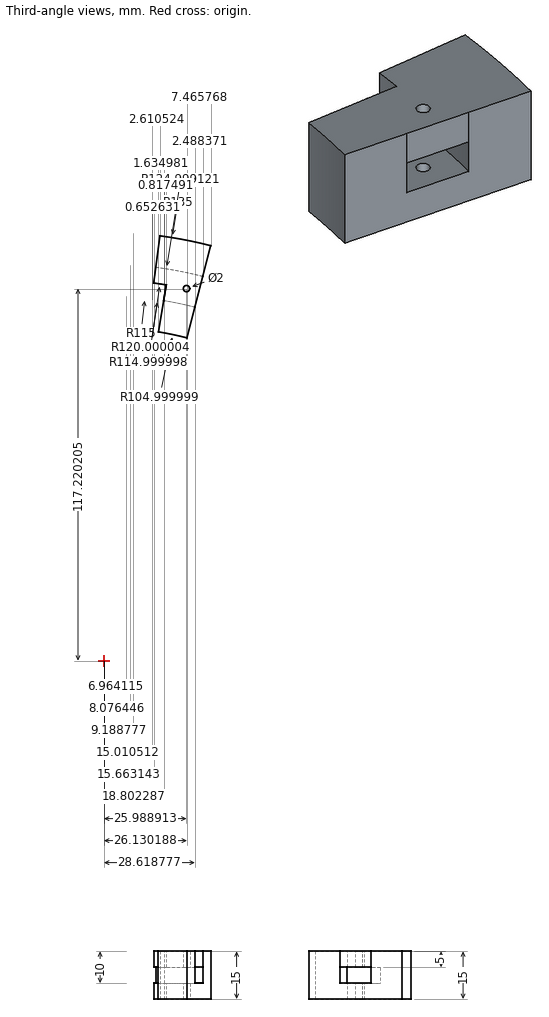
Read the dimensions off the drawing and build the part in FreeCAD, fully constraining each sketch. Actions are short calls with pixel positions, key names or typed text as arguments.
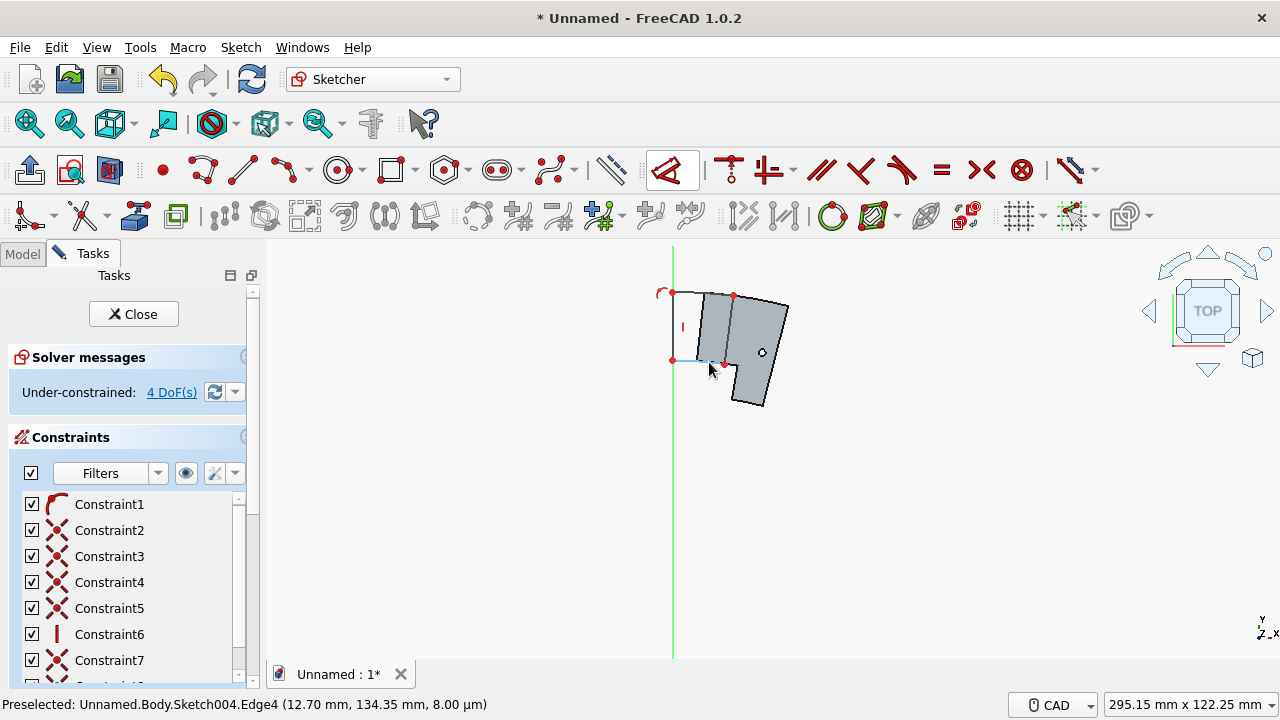
click(709, 362)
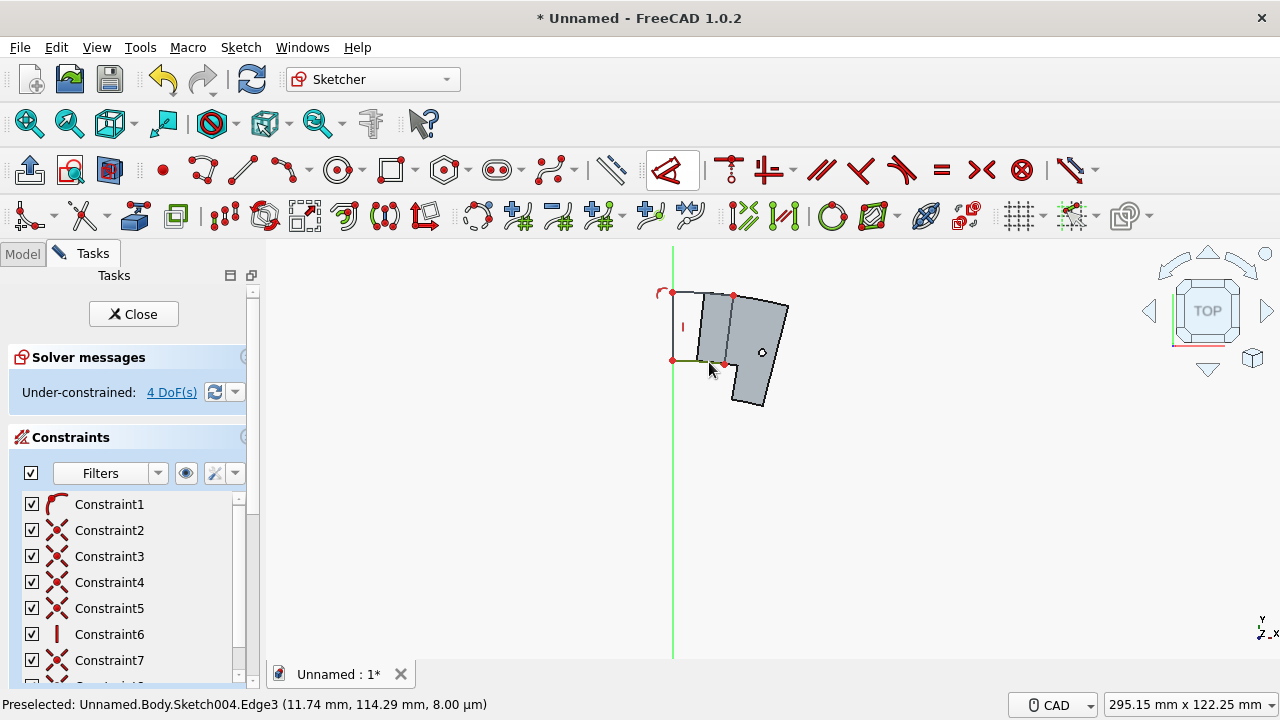
click(694, 170)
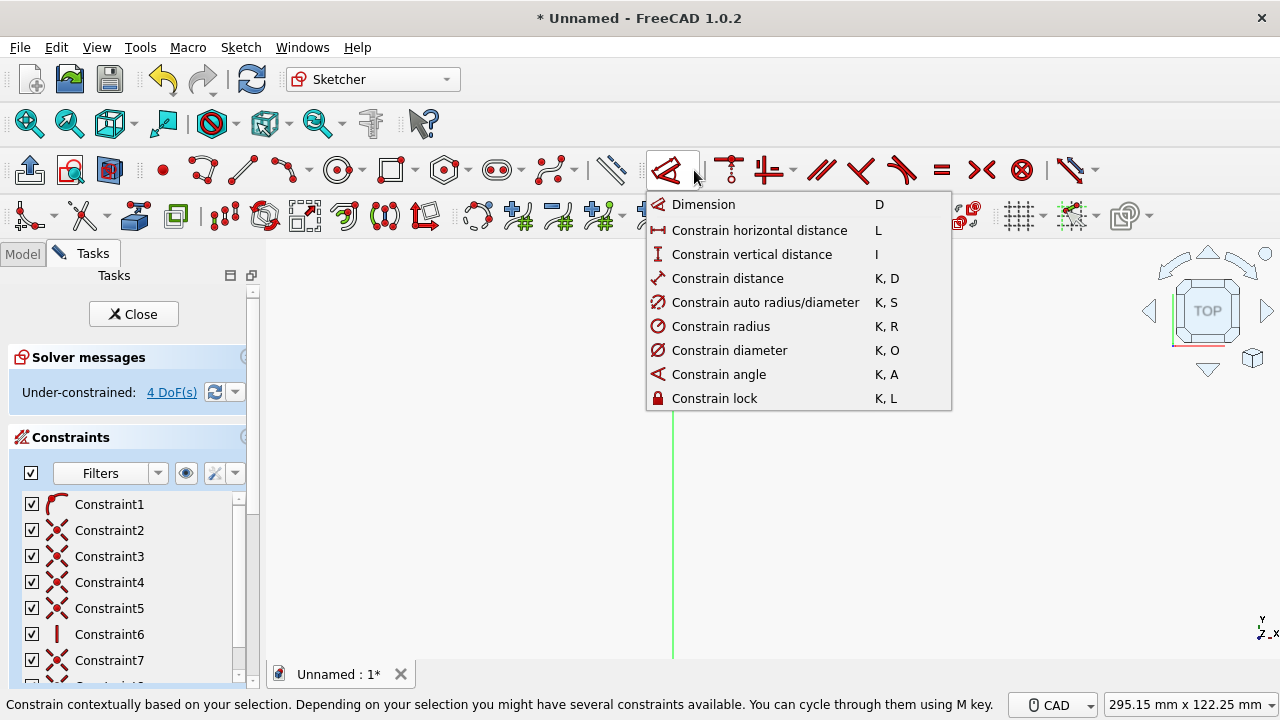
click(799, 326)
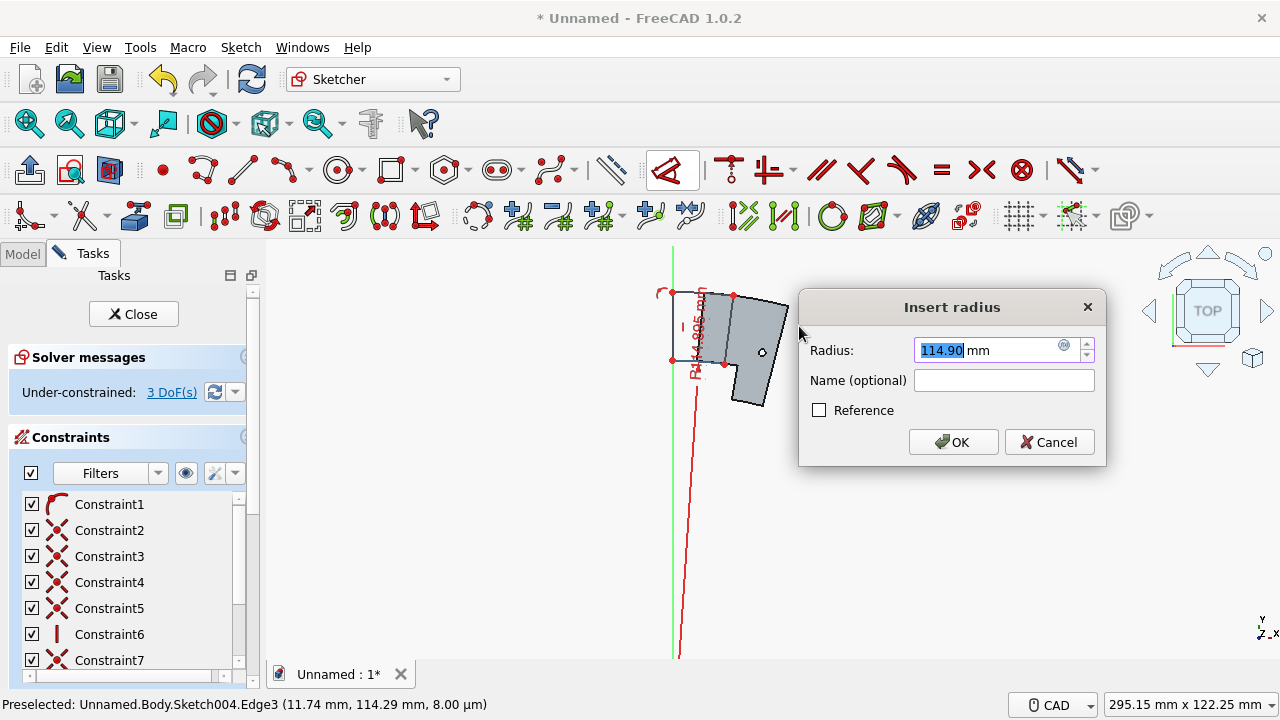
text(115)
key(Return)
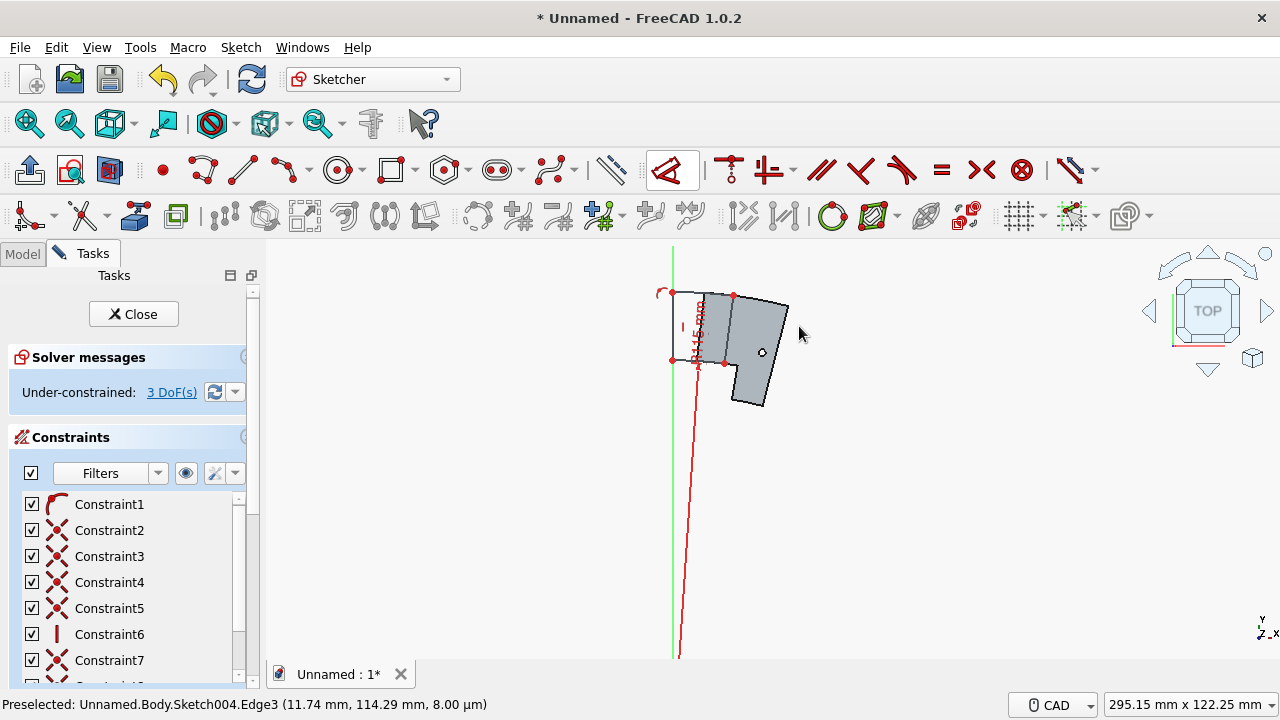
click(715, 294)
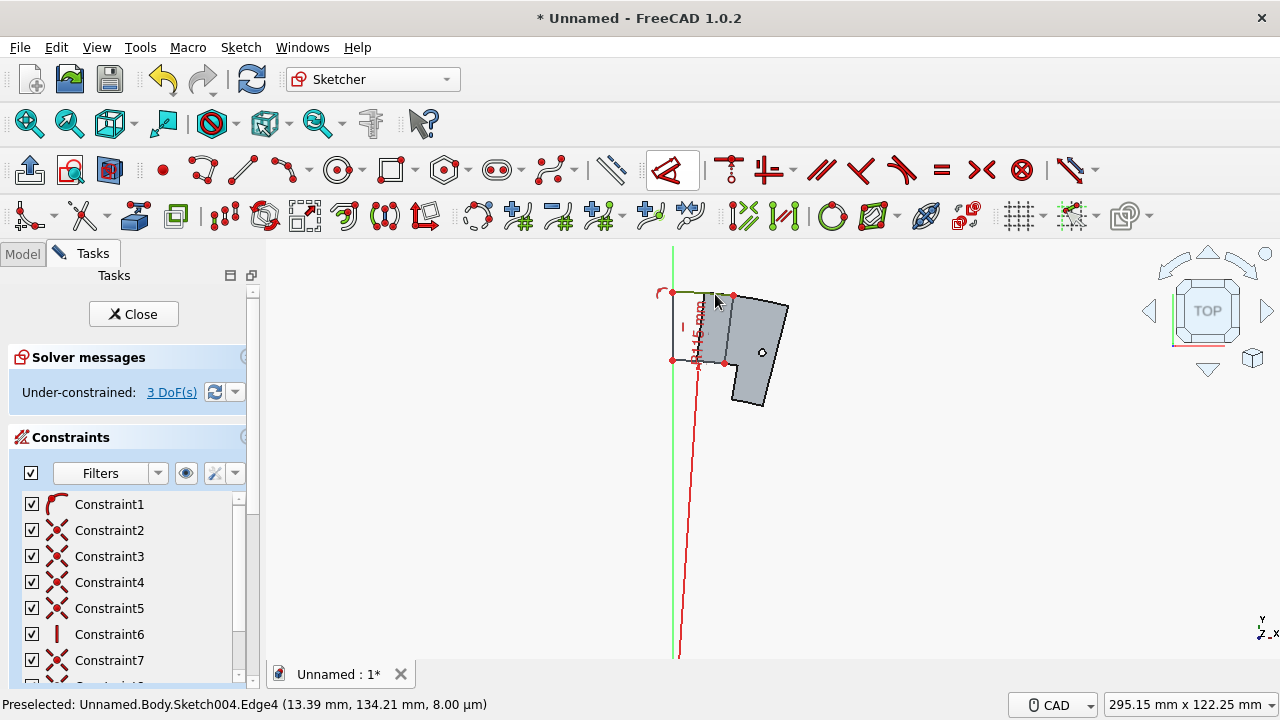
key(k)
key(r)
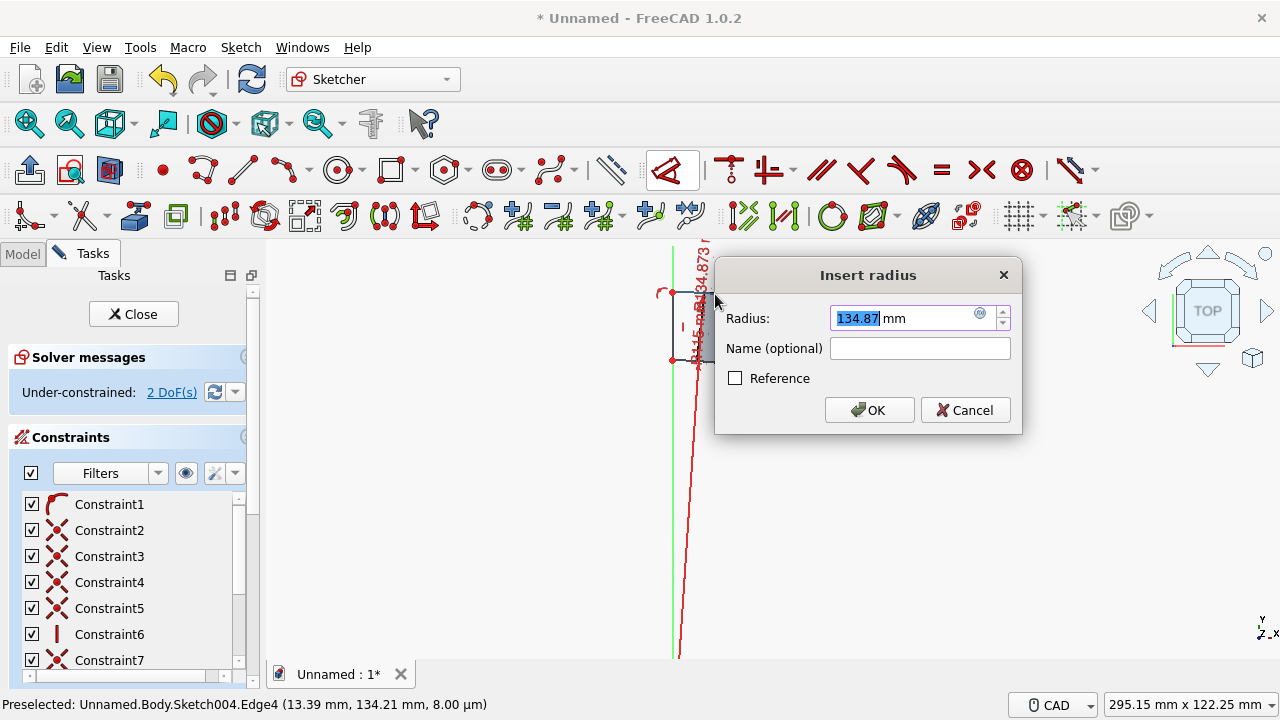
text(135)
key(Return)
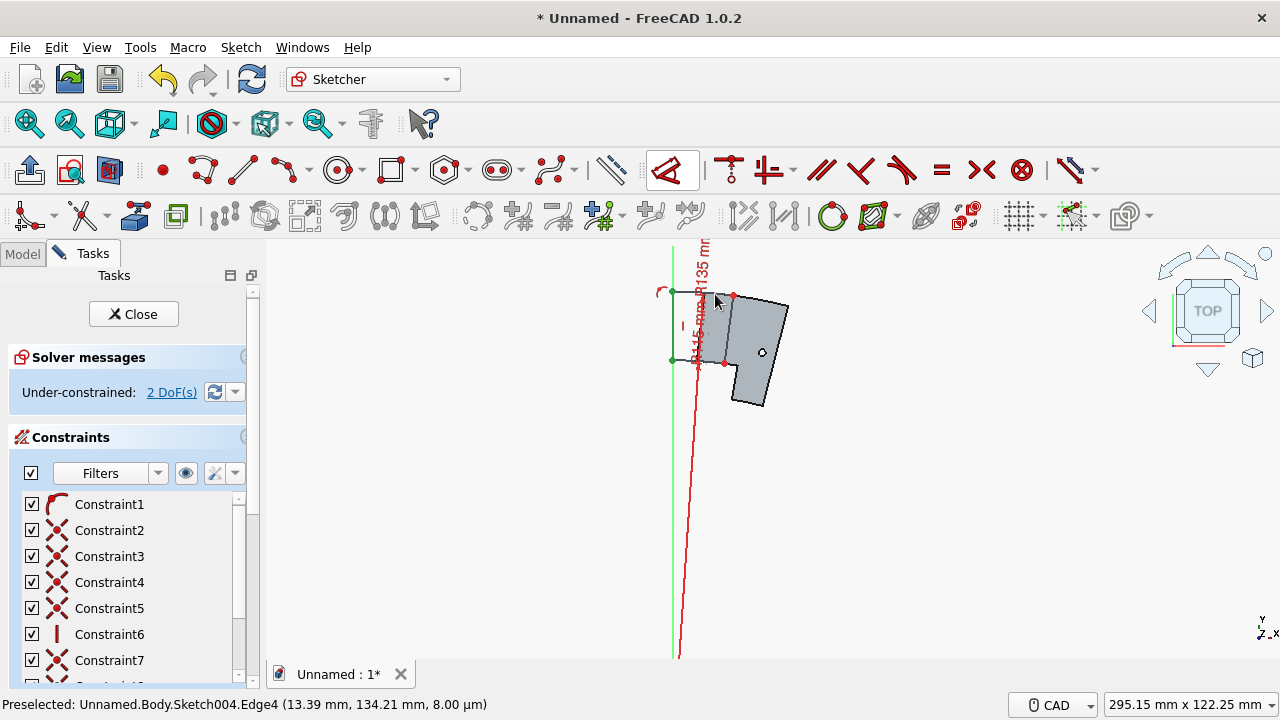
scroll(727, 343, up, 8)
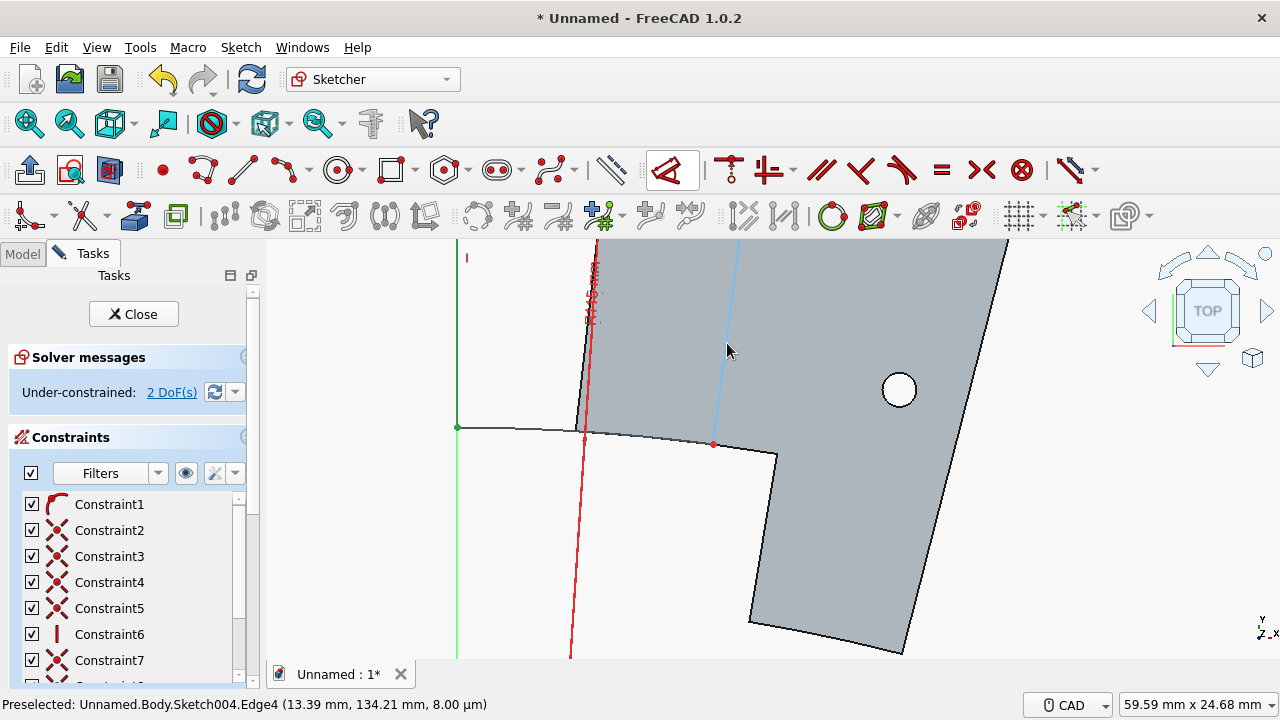
click(726, 343)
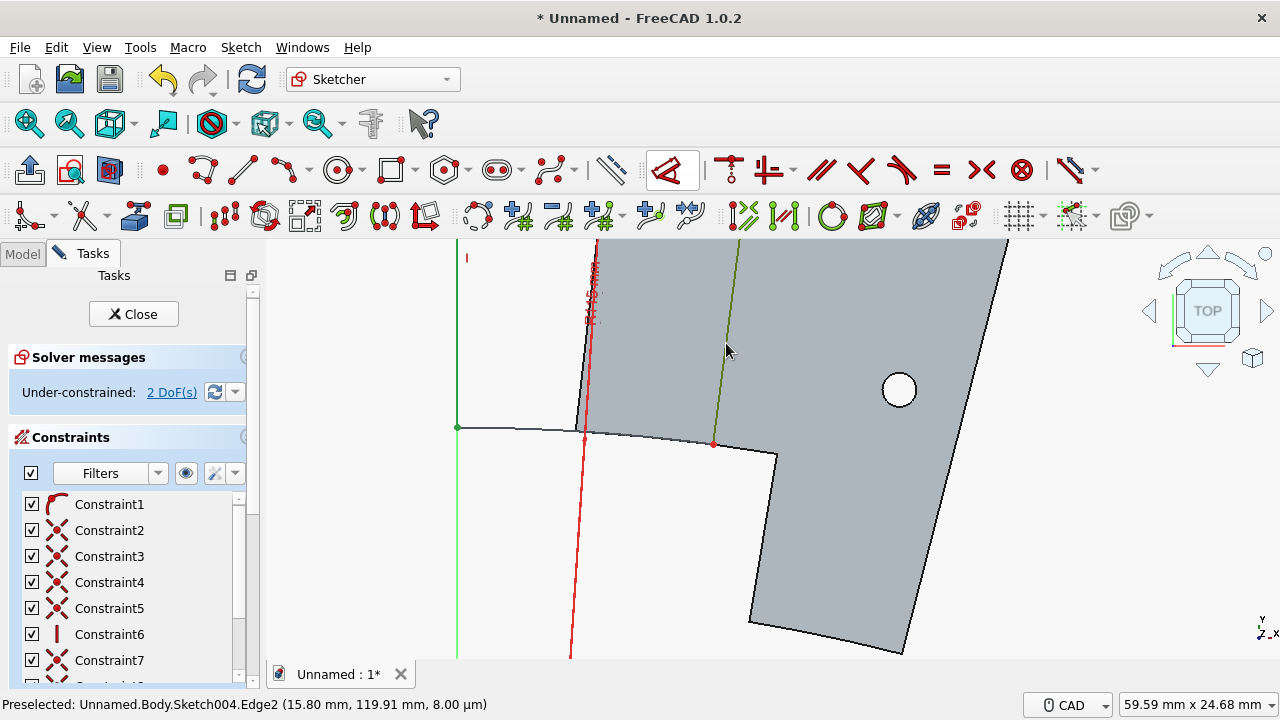
key(l)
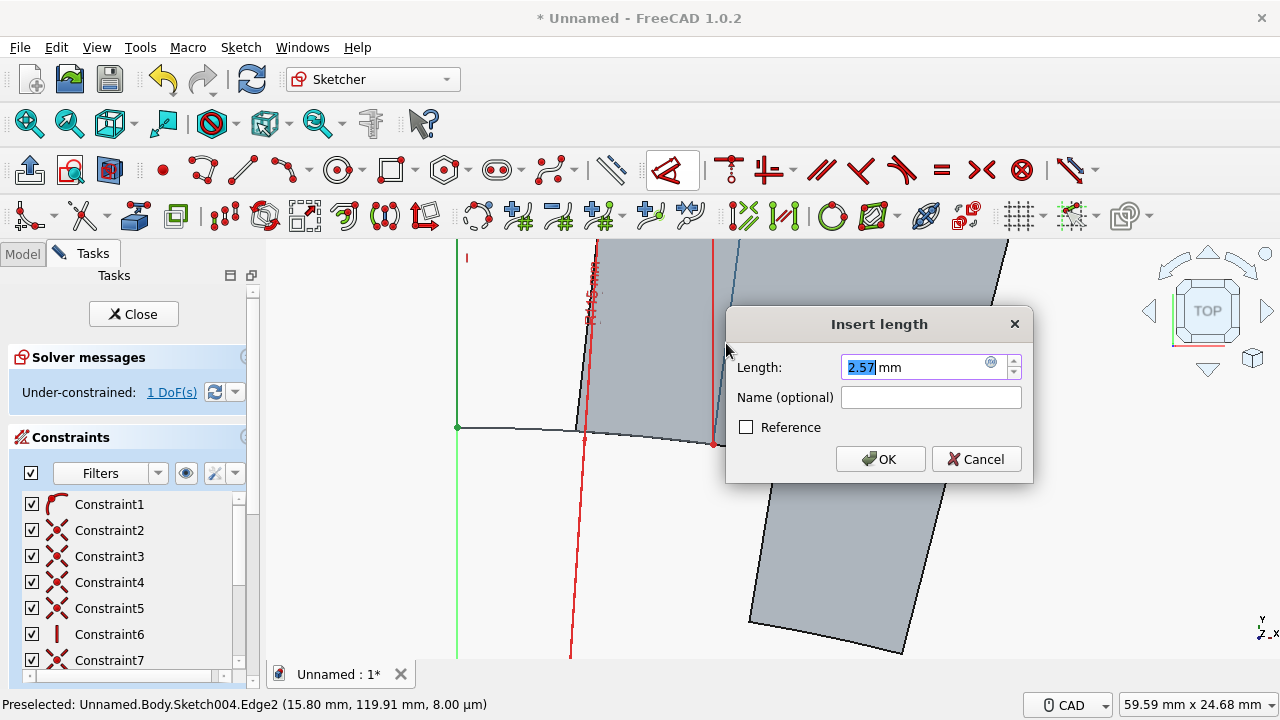
text(2.610524)
key(Return)